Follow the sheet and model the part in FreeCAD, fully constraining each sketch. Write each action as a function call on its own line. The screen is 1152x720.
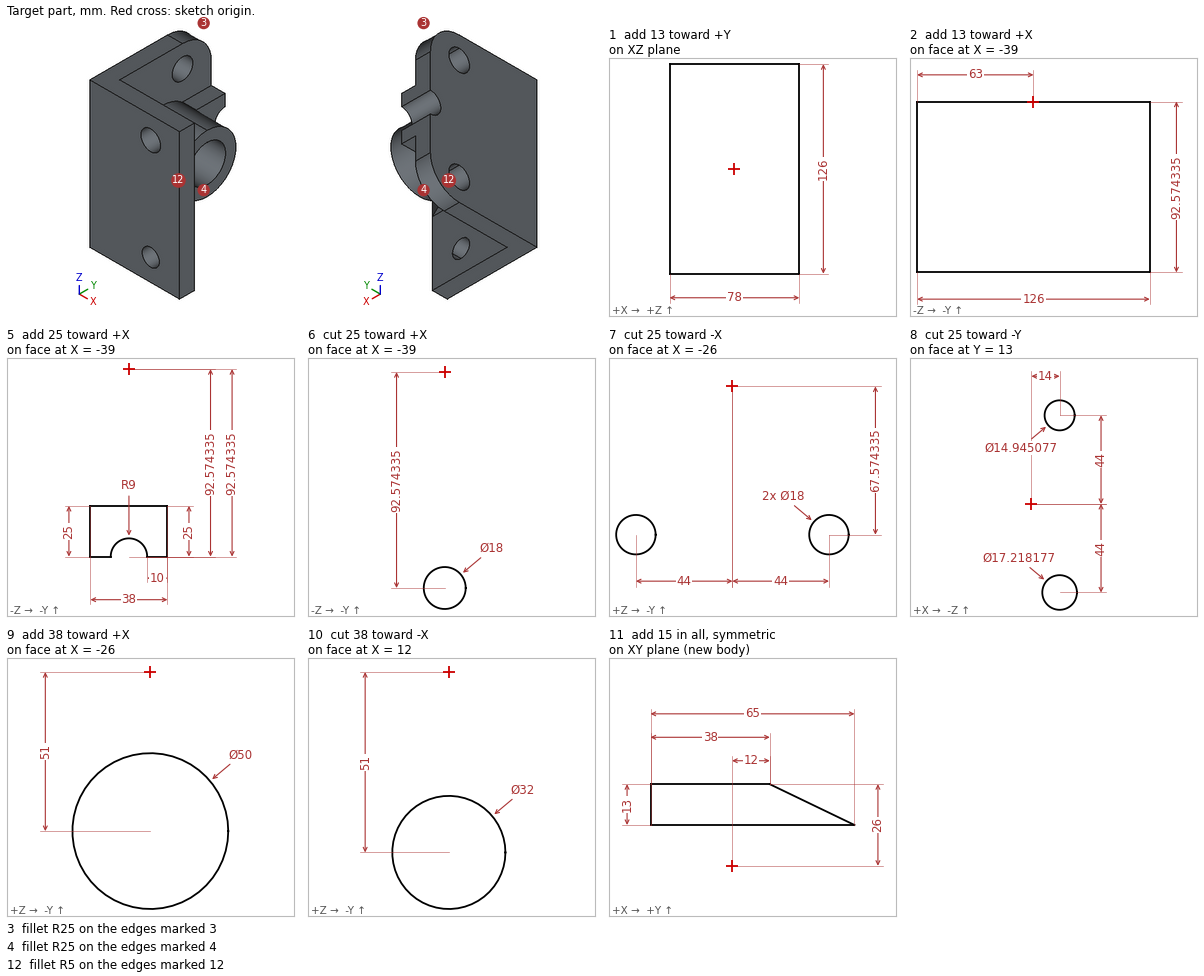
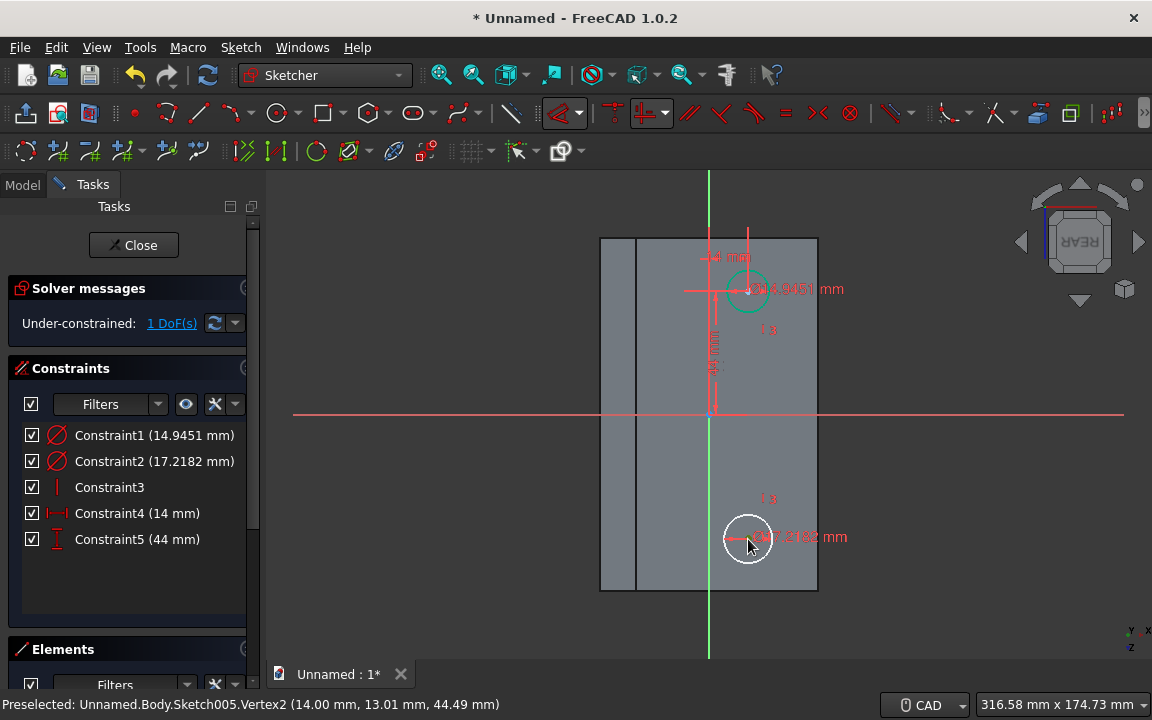
key(i)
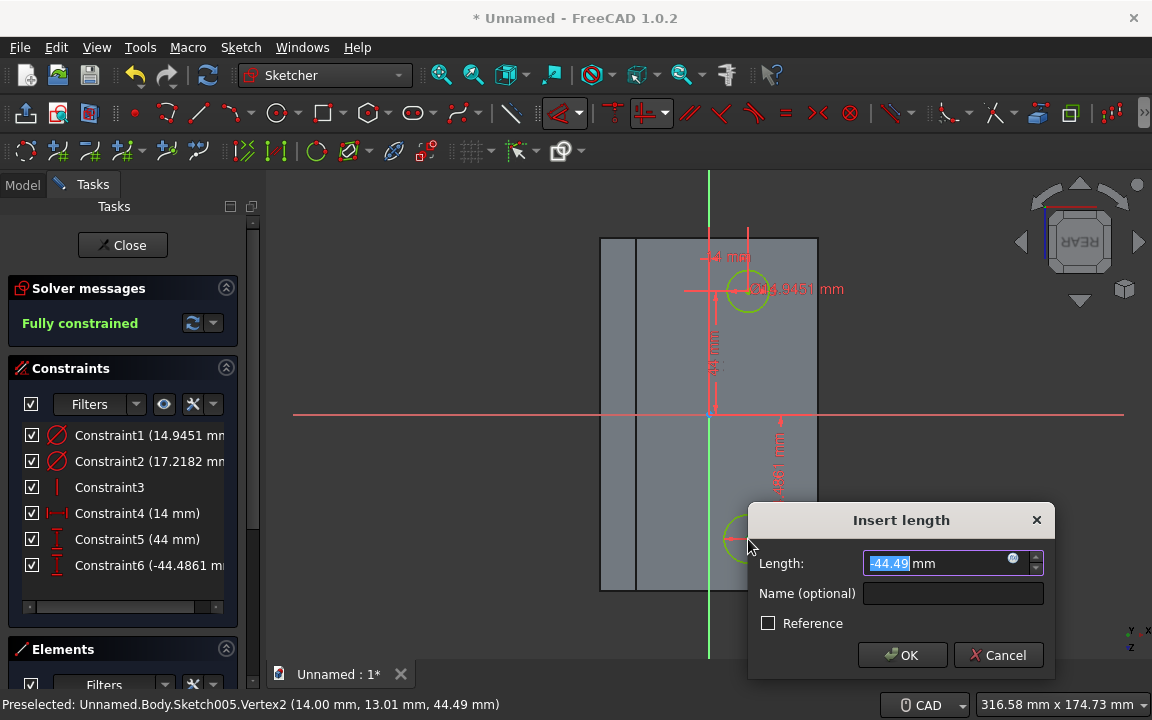
text(-44)
key(Return)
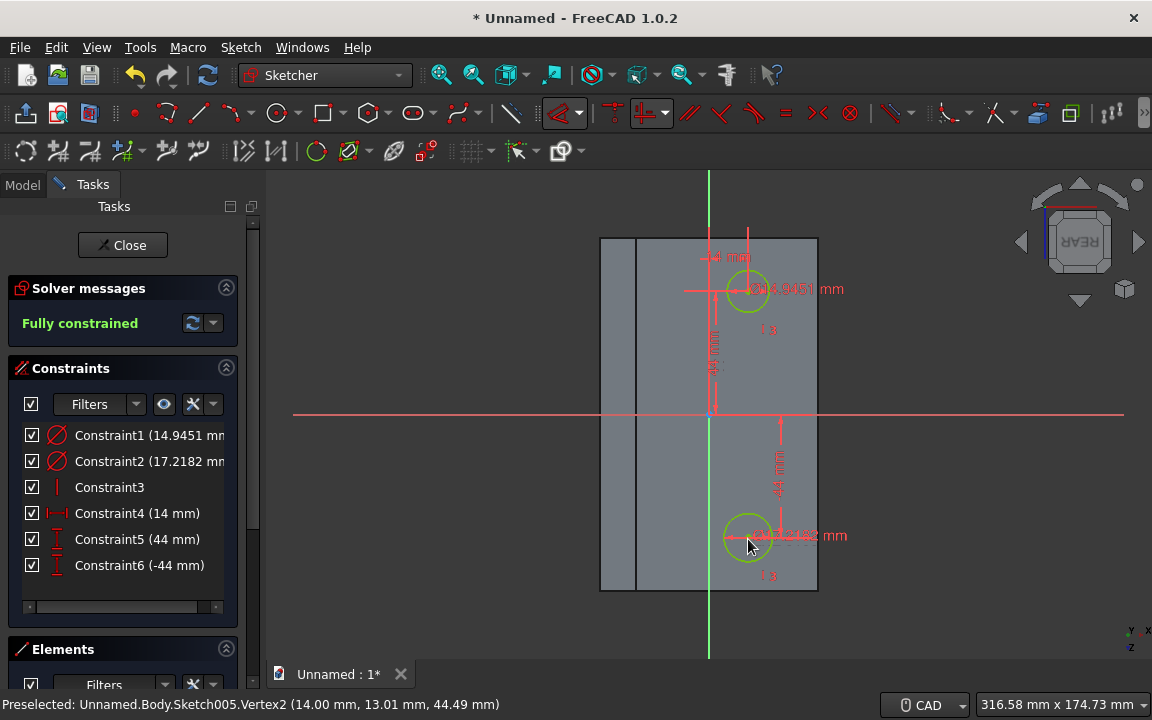
click(123, 245)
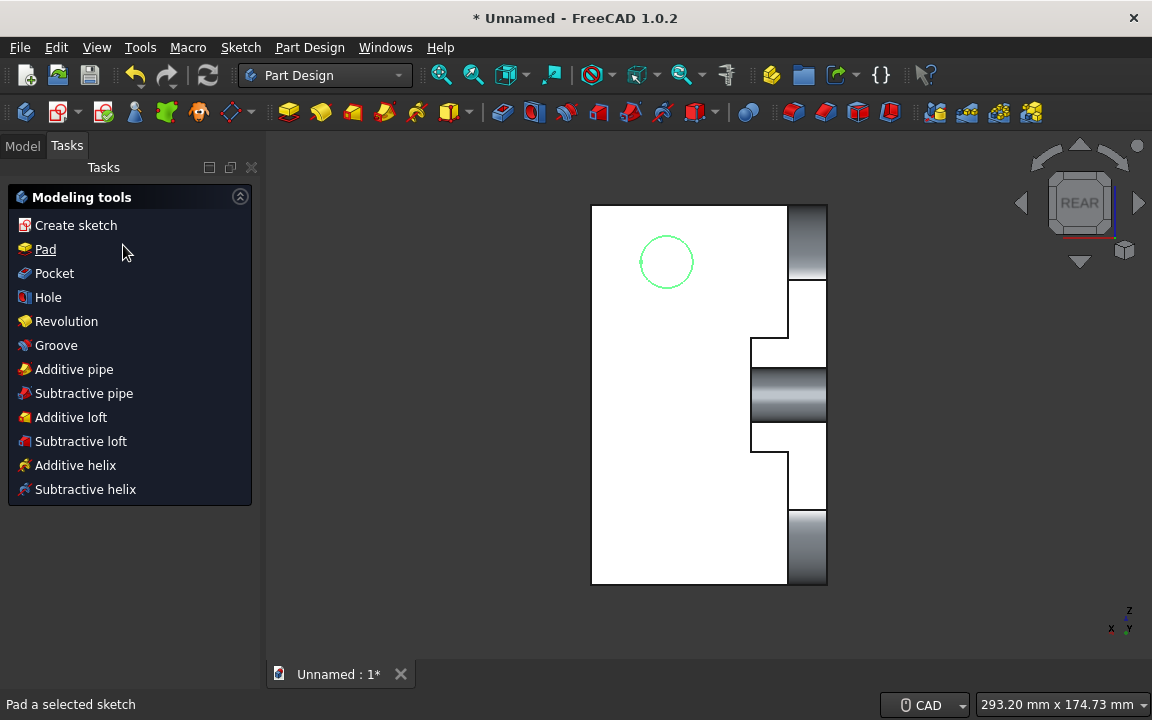
click(504, 112)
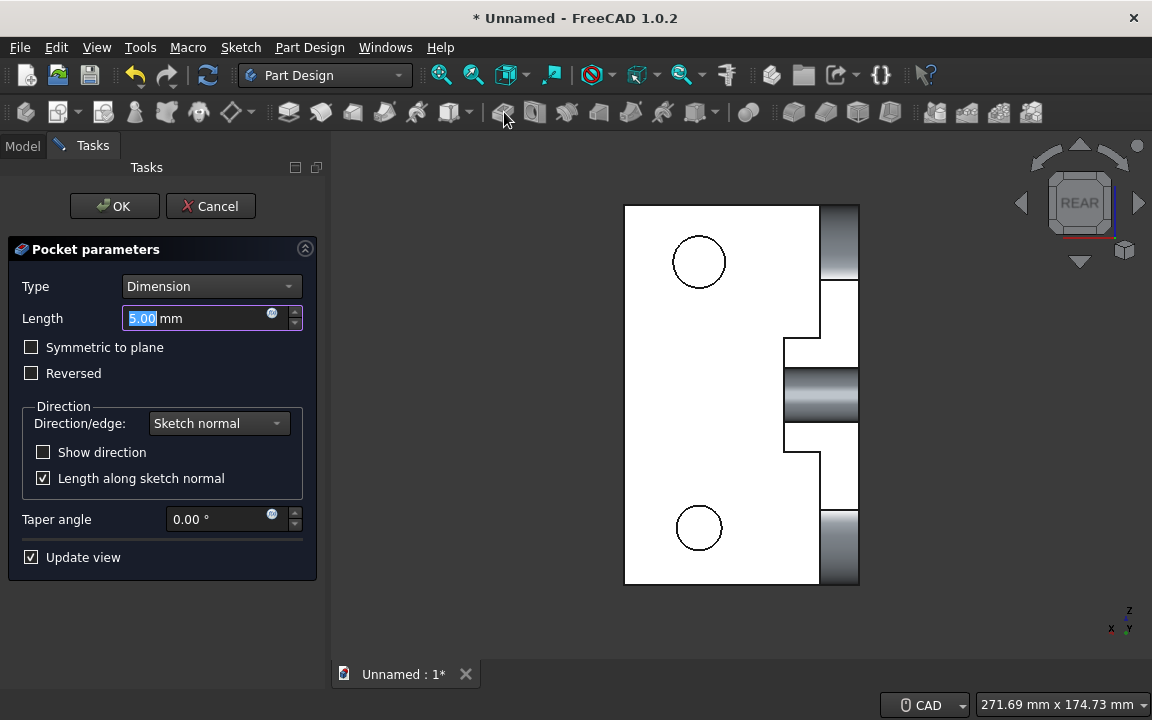
text(25)
key(Tab)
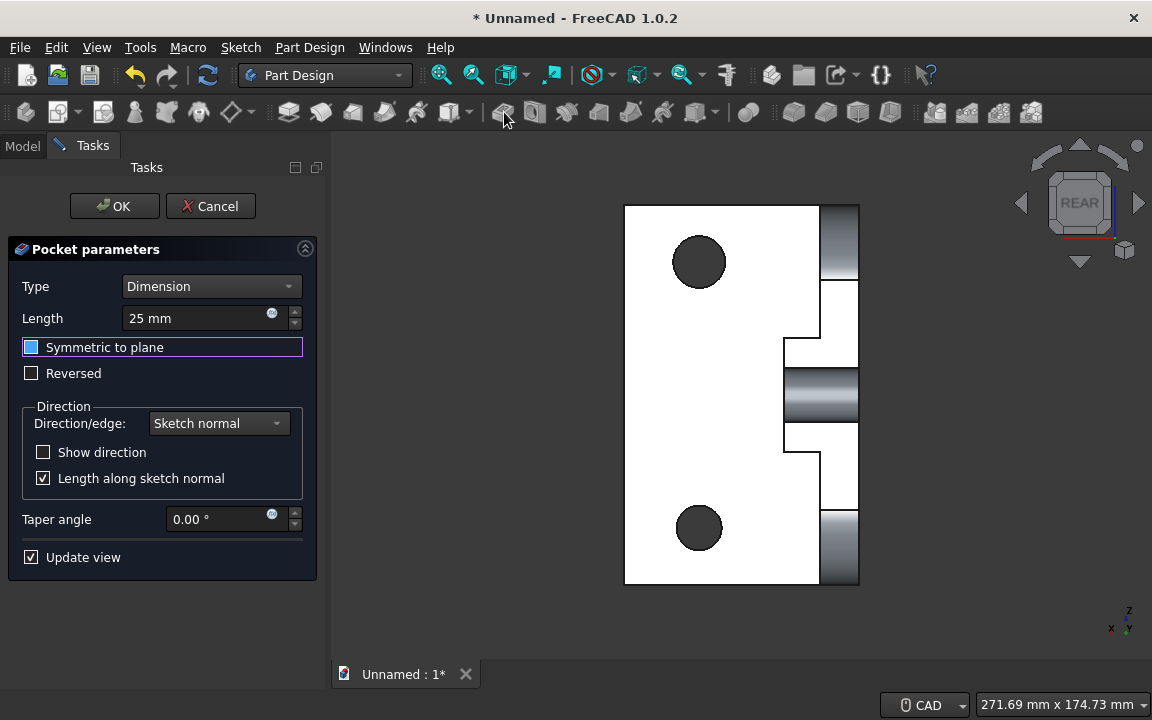
click(115, 206)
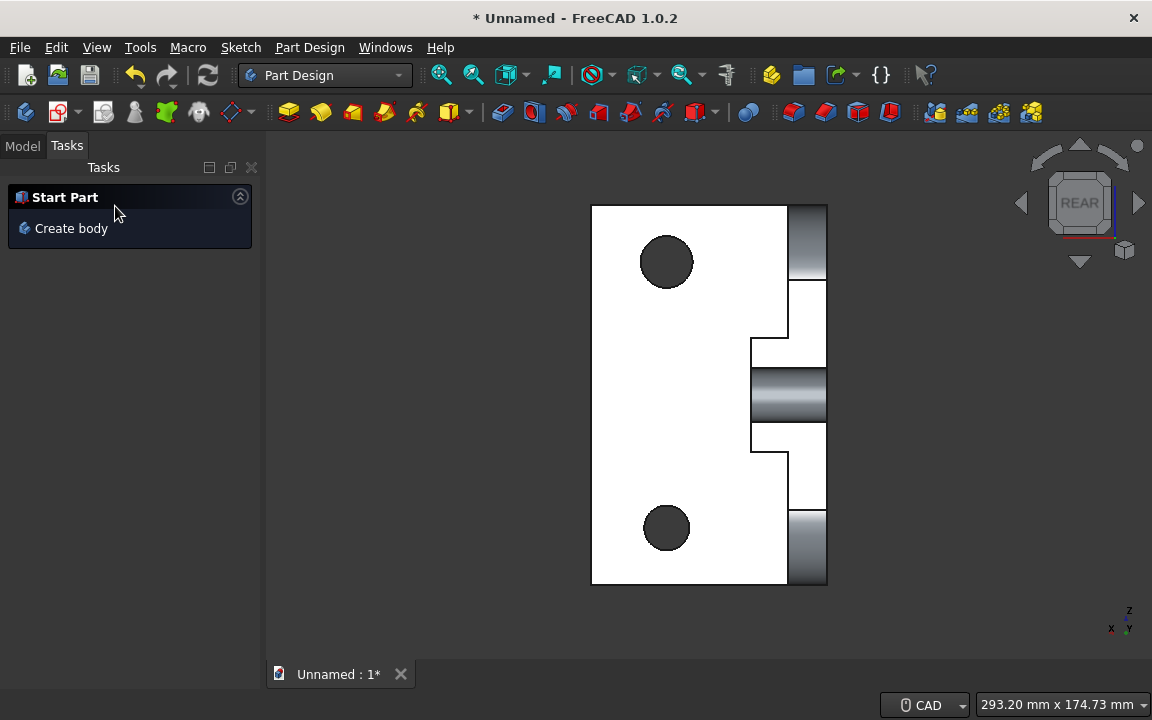
key(0)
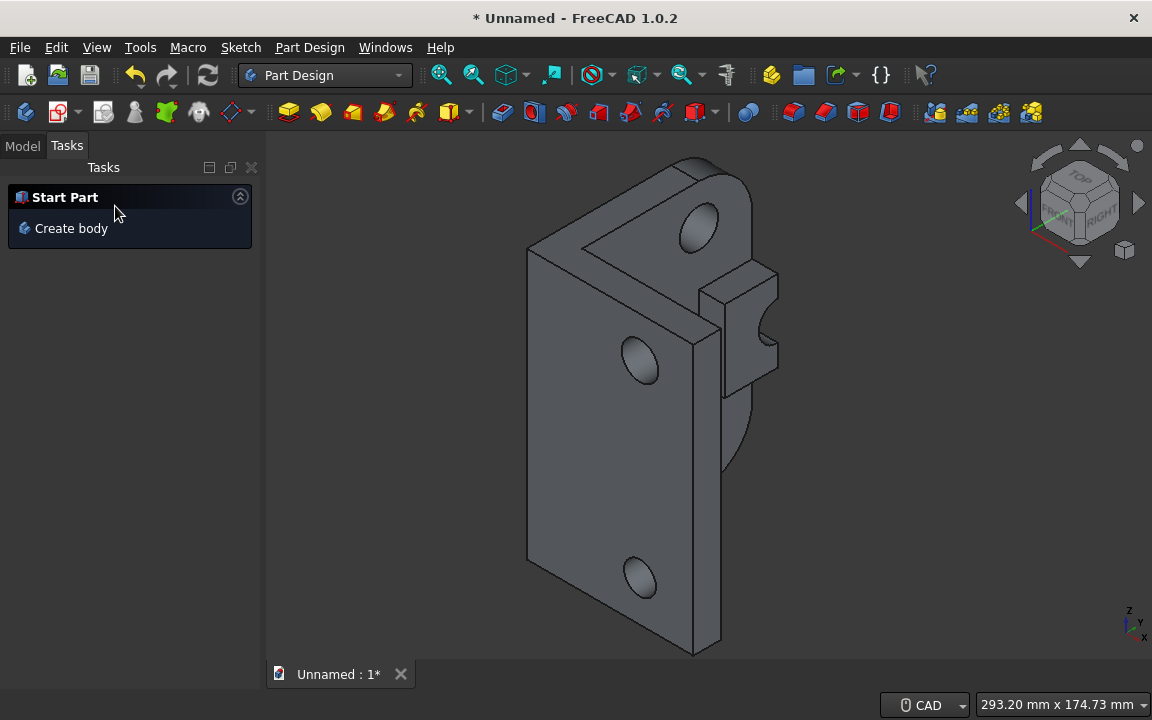
key(3)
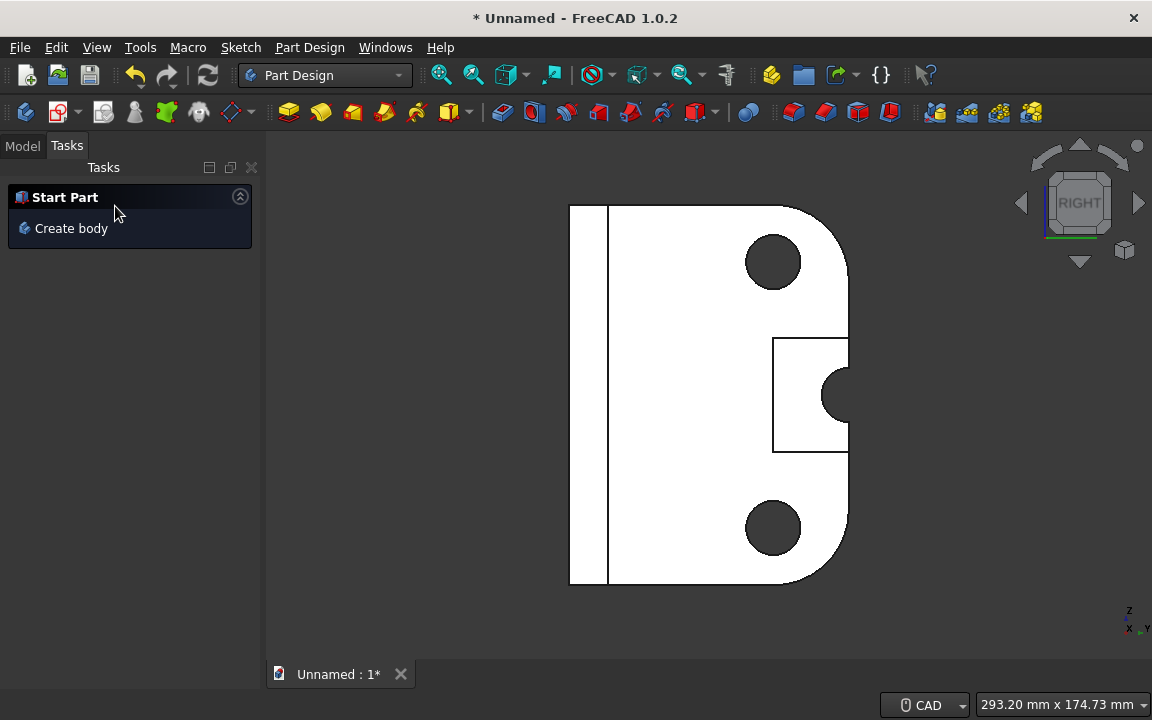
click(694, 448)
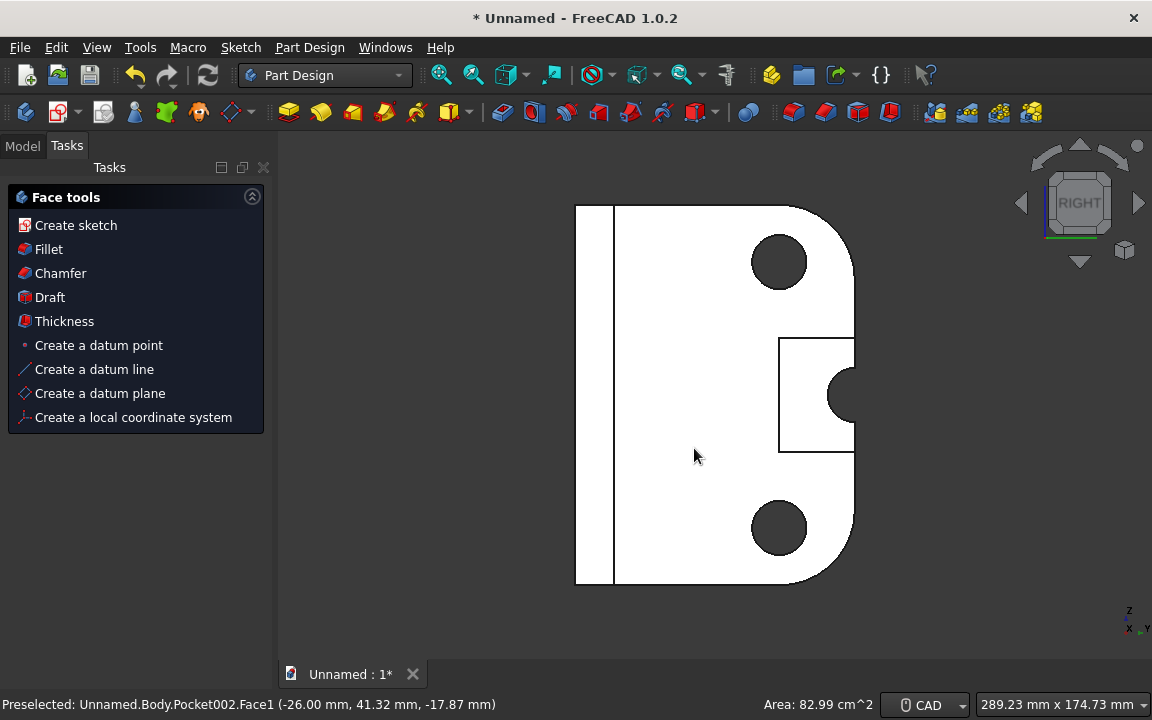
click(58, 112)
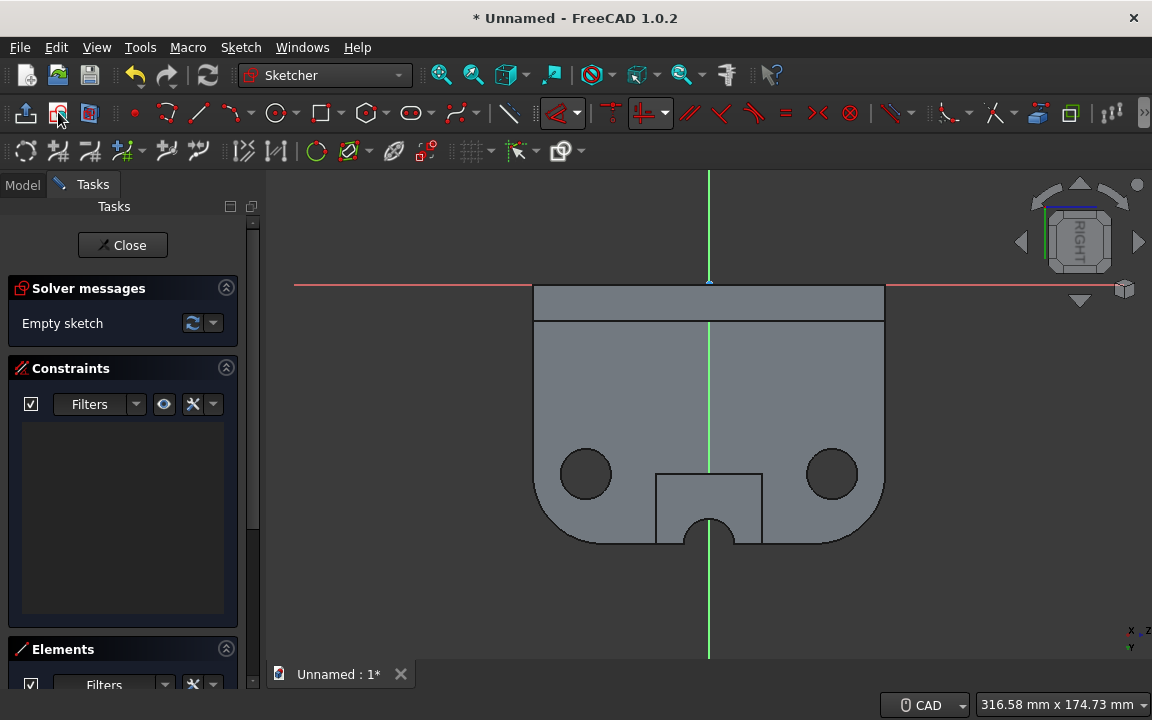
key(q)
key(s)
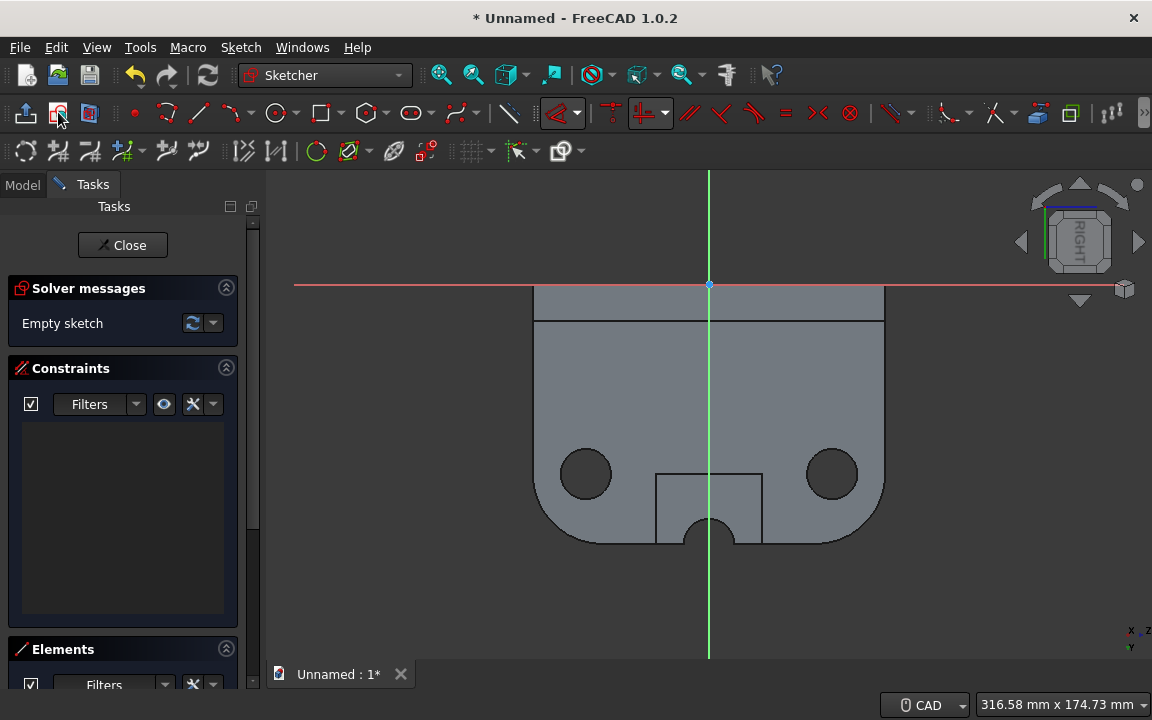
scroll(848, 344, up, 2)